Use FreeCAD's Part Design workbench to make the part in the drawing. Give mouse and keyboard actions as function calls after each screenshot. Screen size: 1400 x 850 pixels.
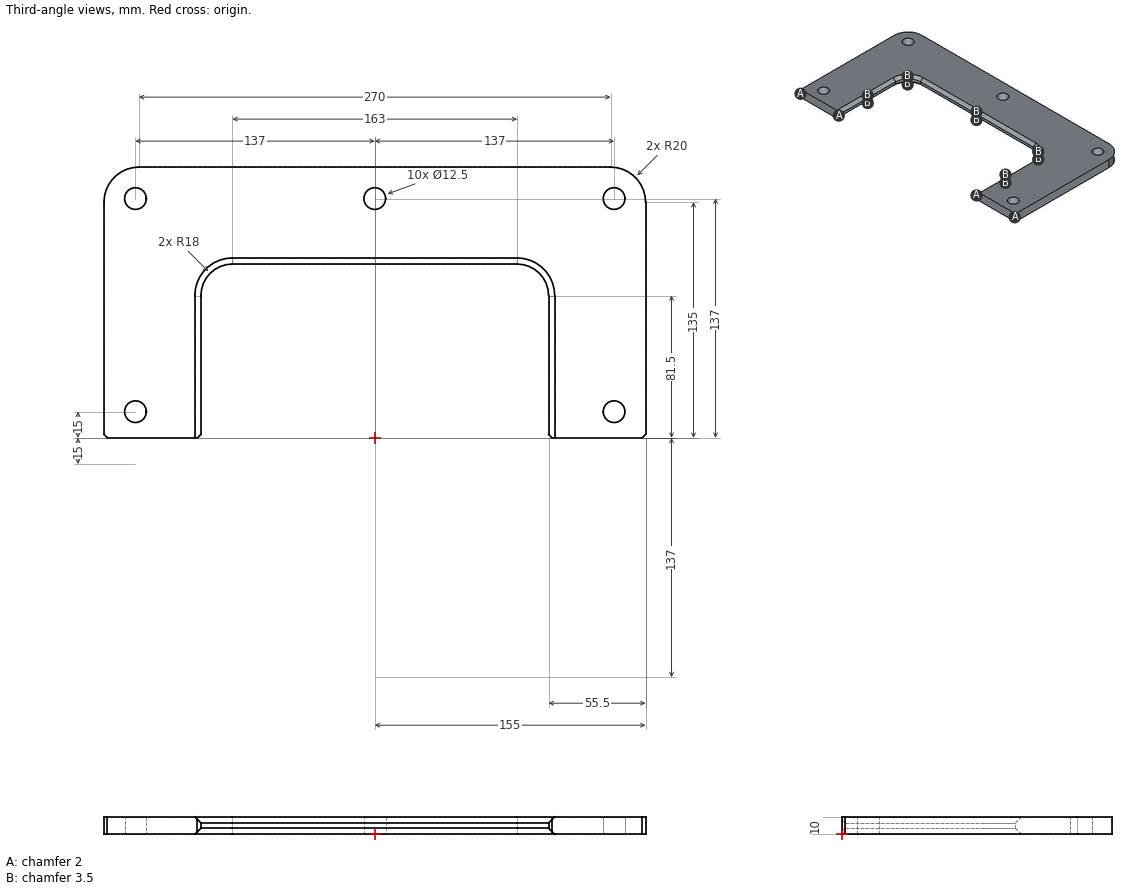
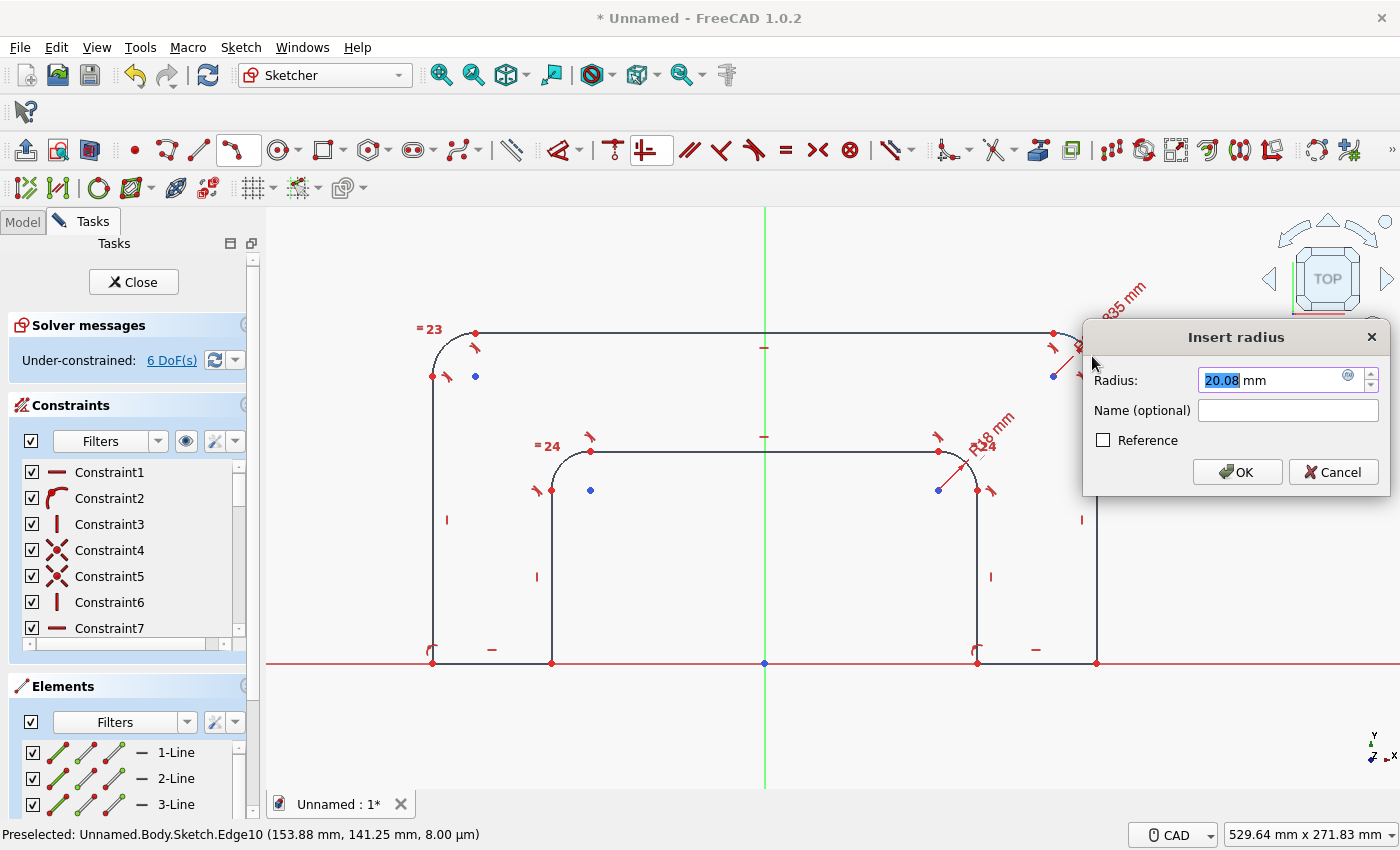
text(20)
key(Return)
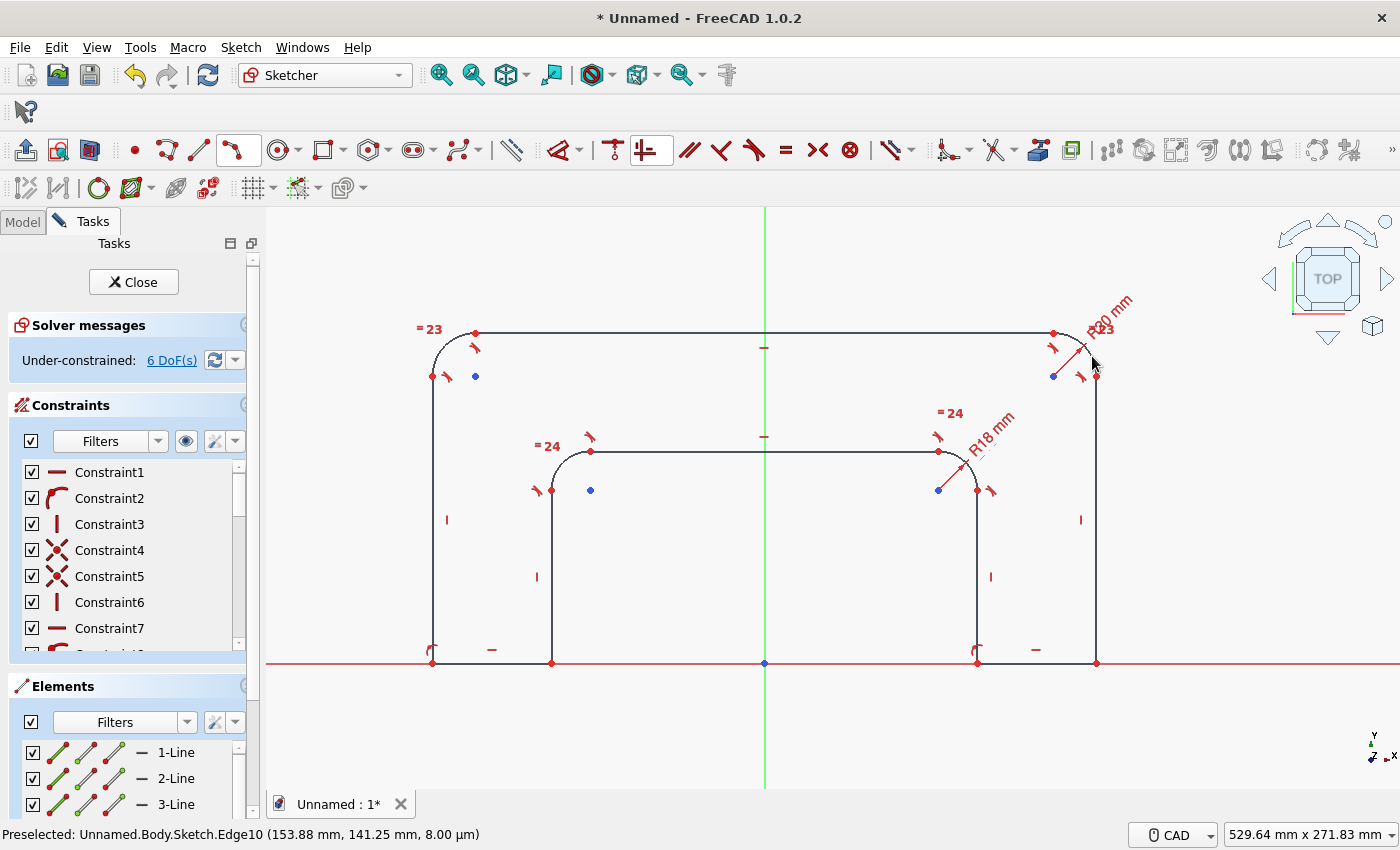
click(695, 452)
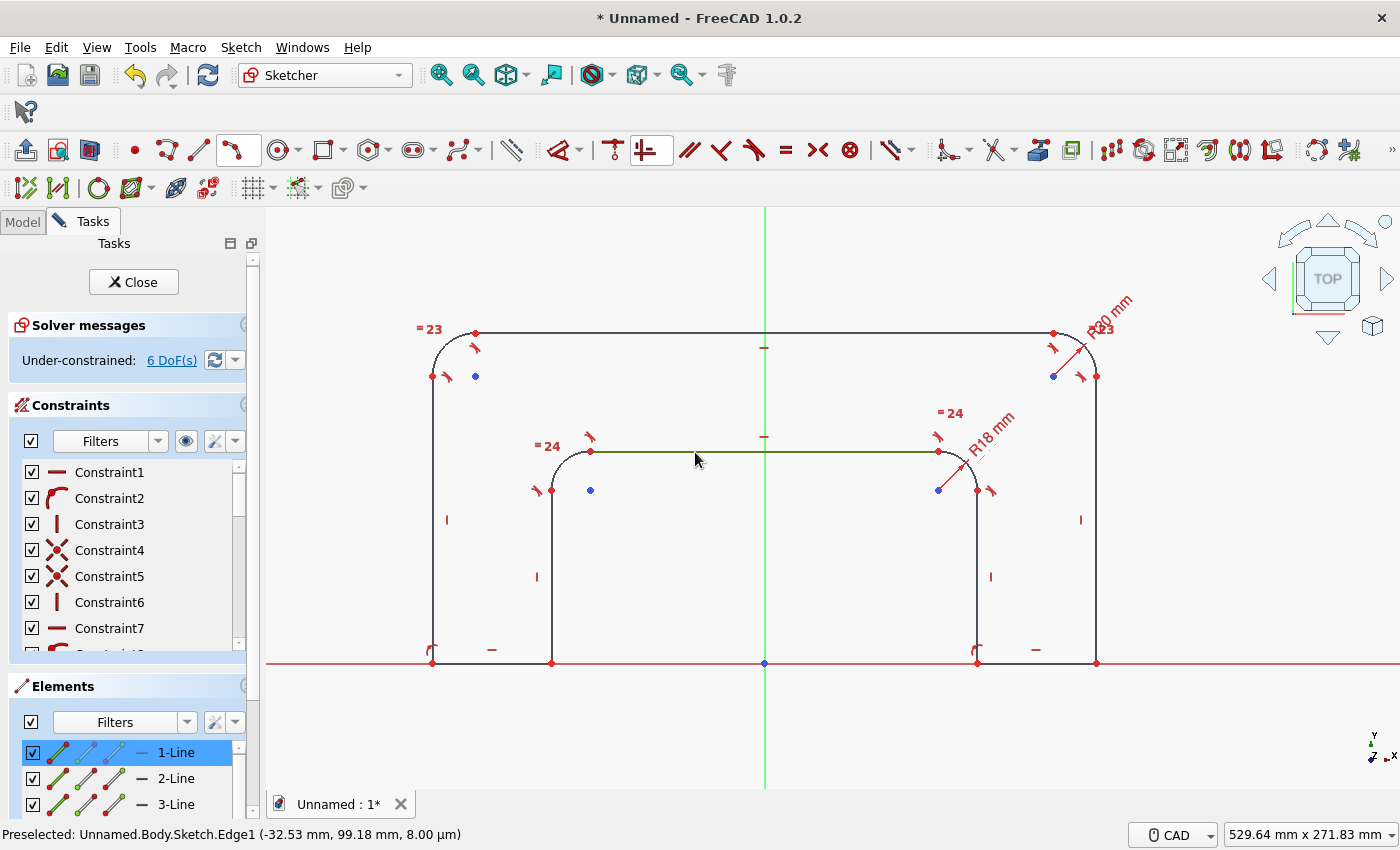
key(l)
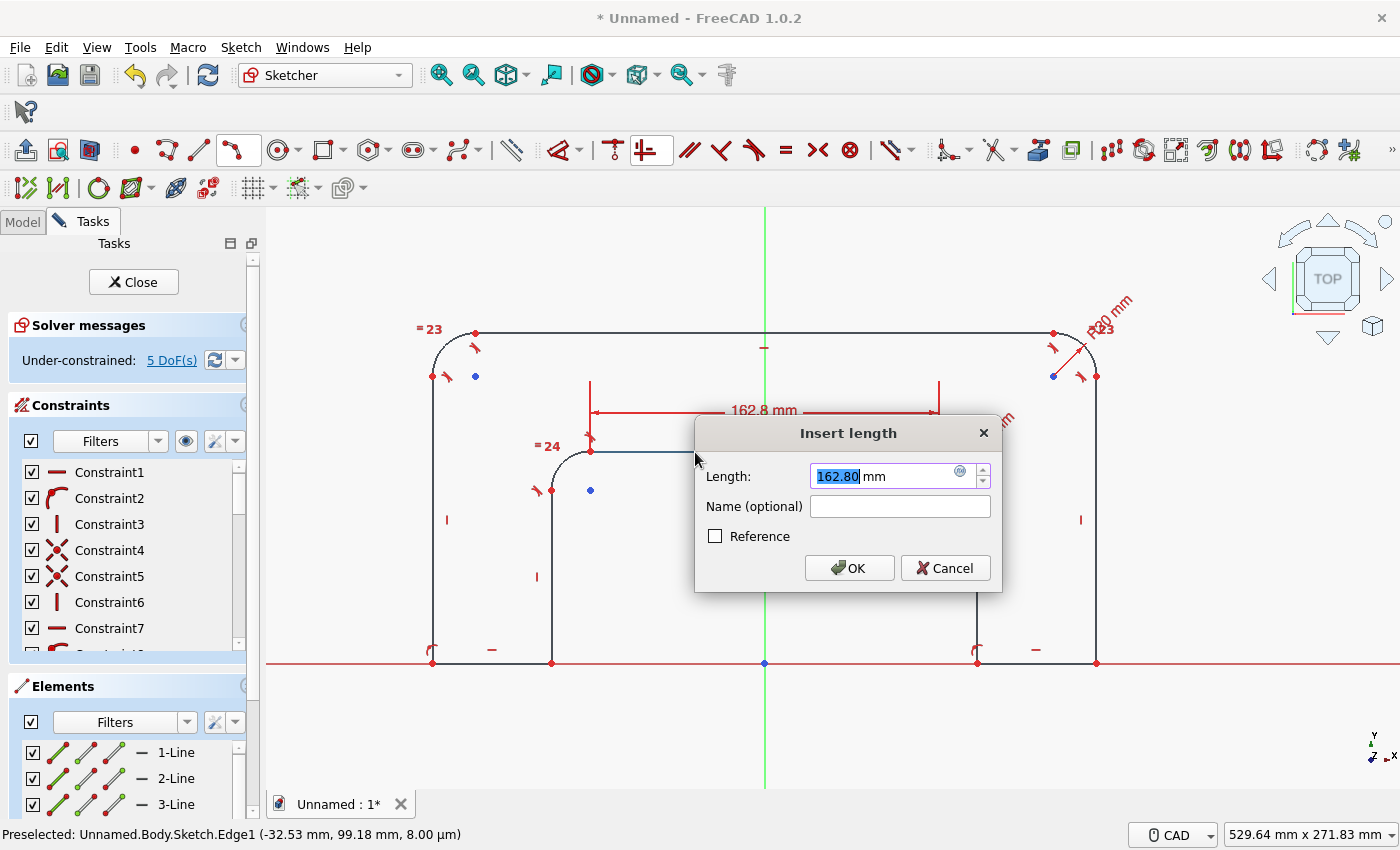
text(163)
key(Return)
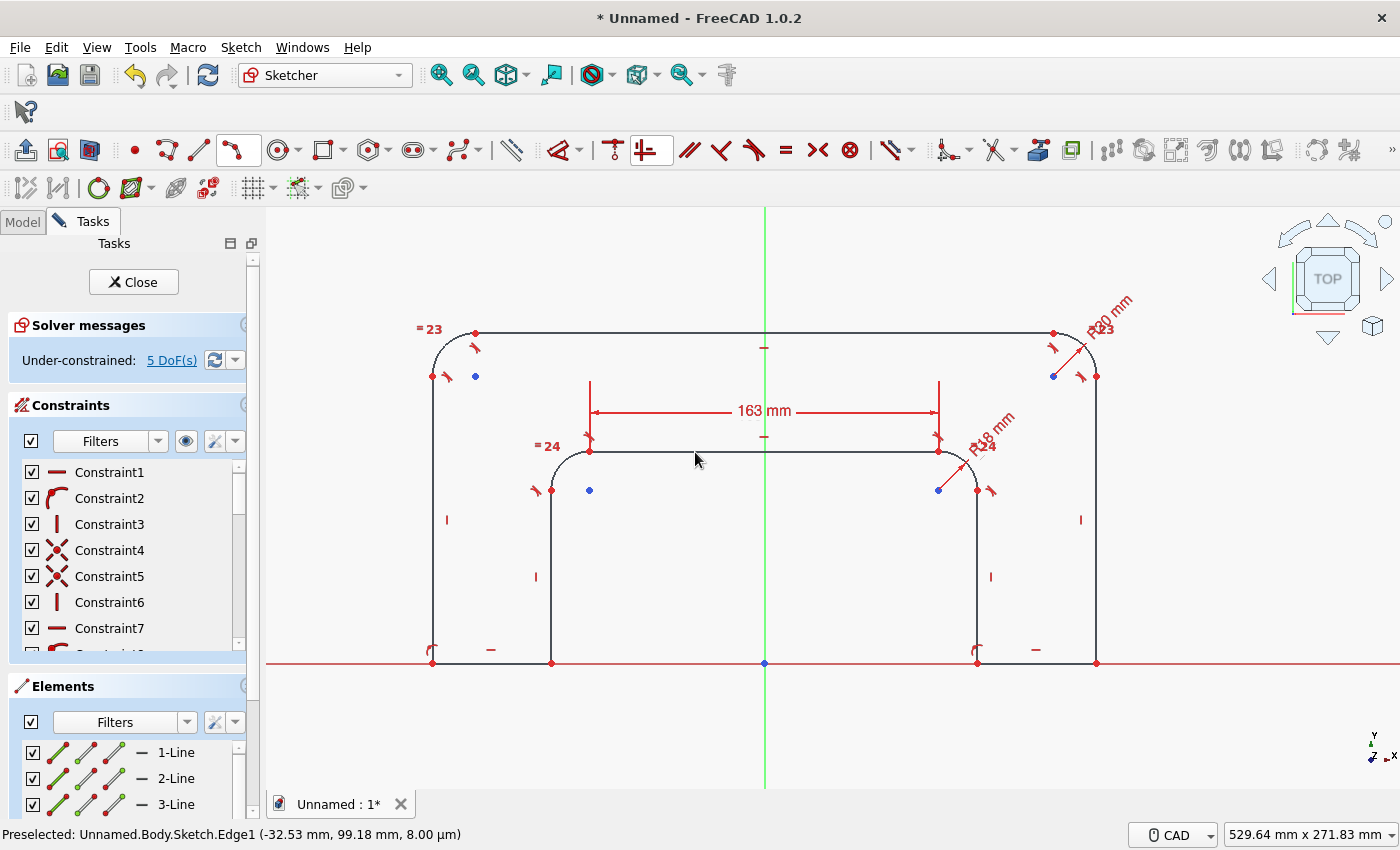
click(1096, 578)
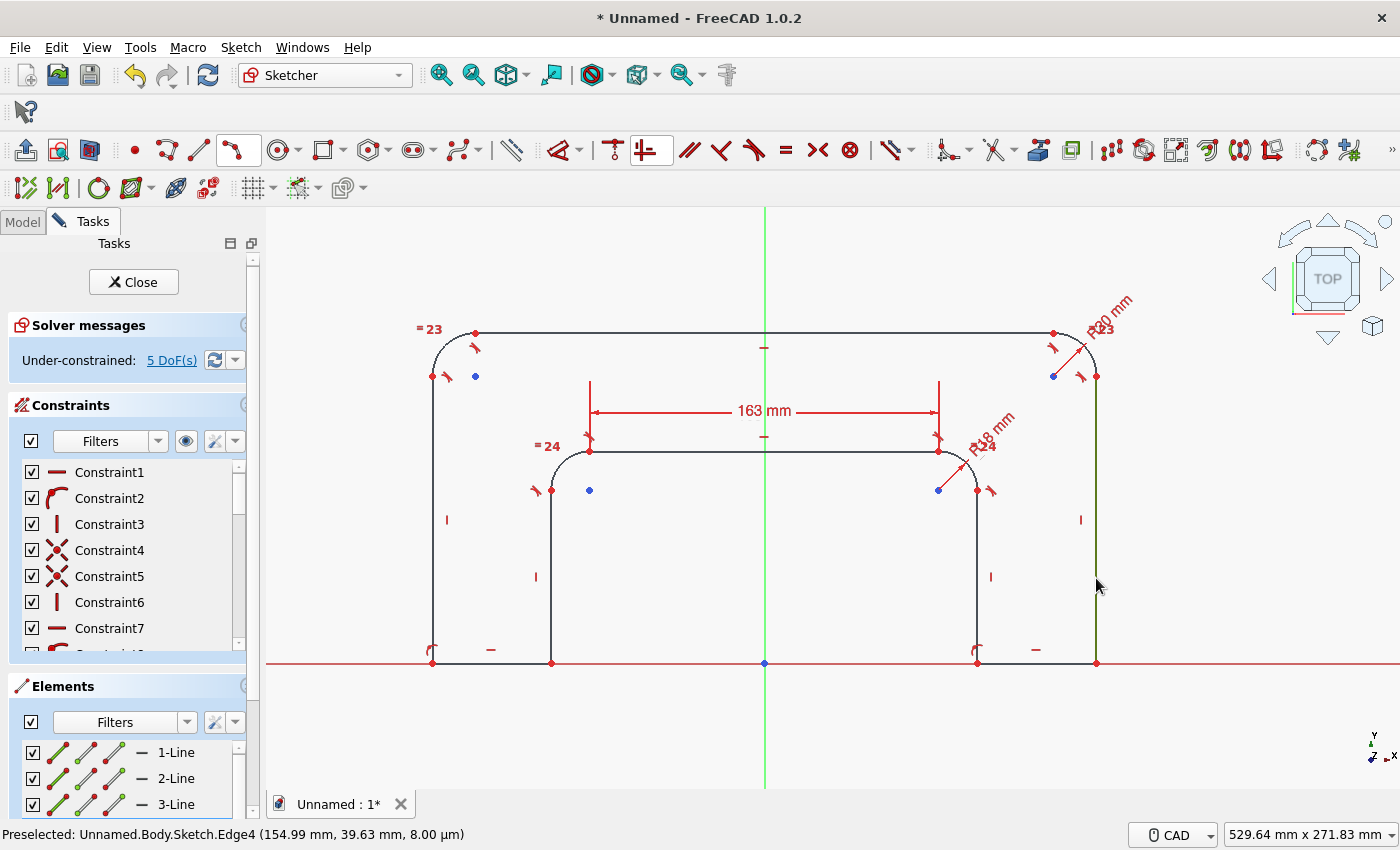
key(i)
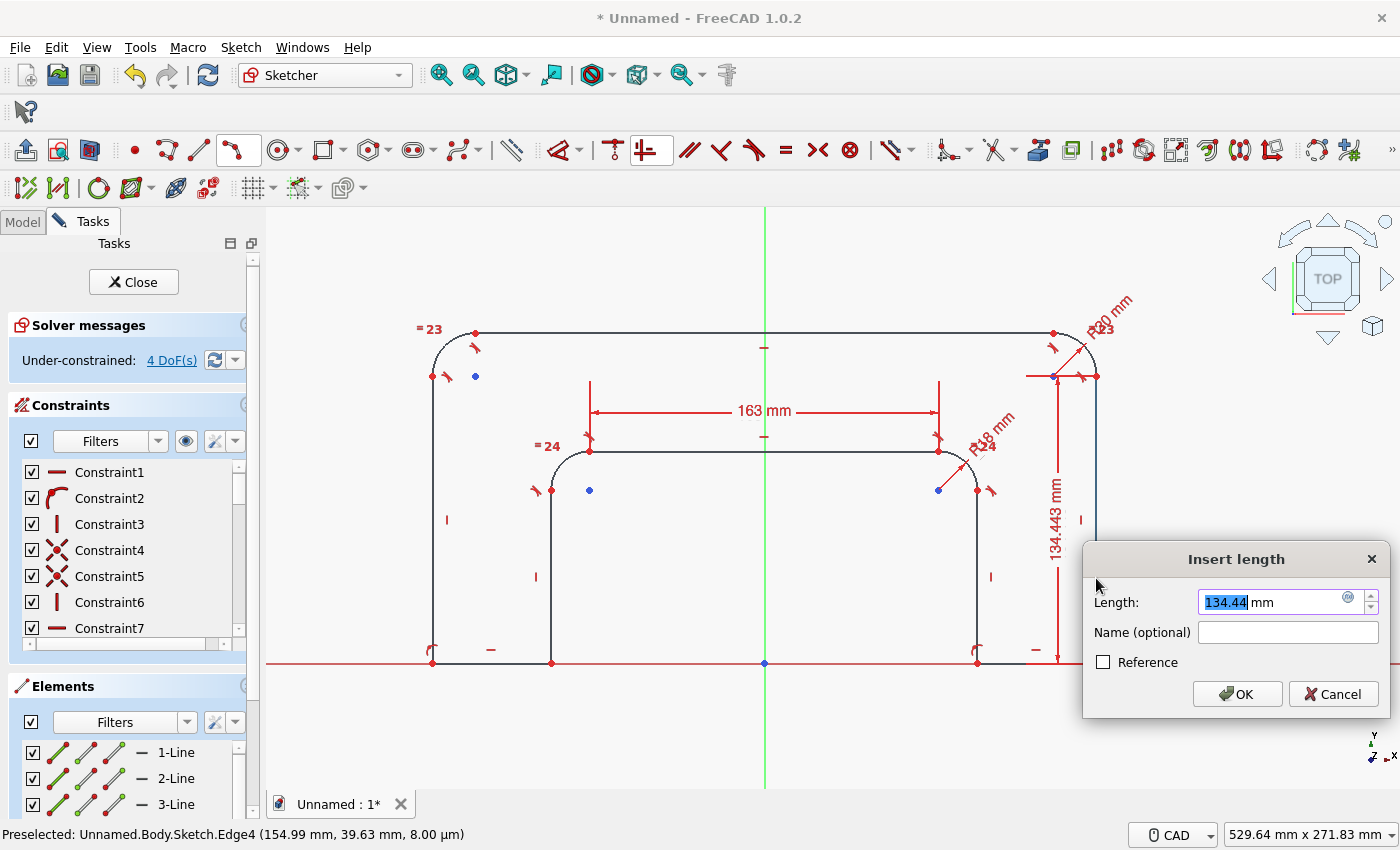
text(135)
key(Return)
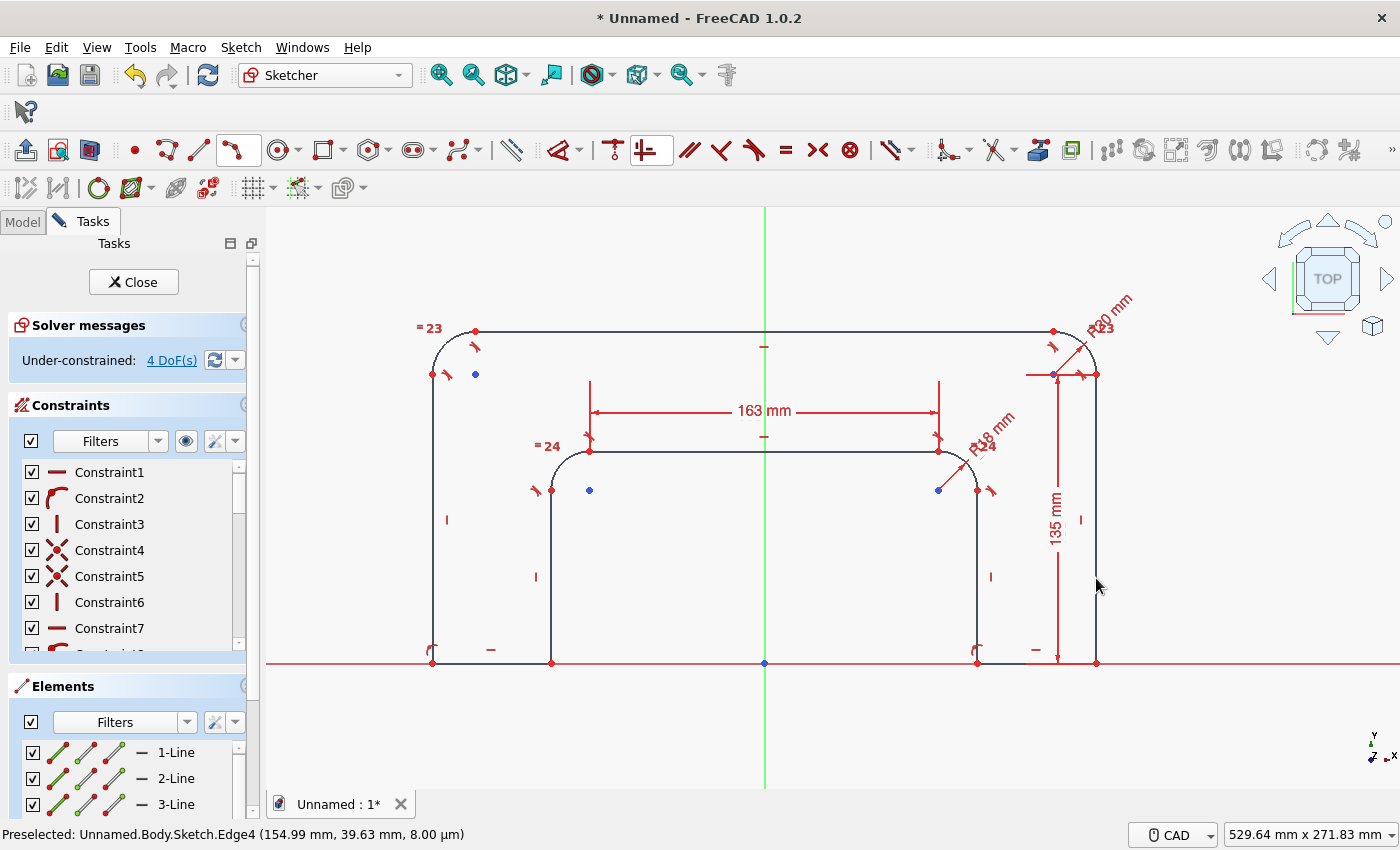
click(880, 332)